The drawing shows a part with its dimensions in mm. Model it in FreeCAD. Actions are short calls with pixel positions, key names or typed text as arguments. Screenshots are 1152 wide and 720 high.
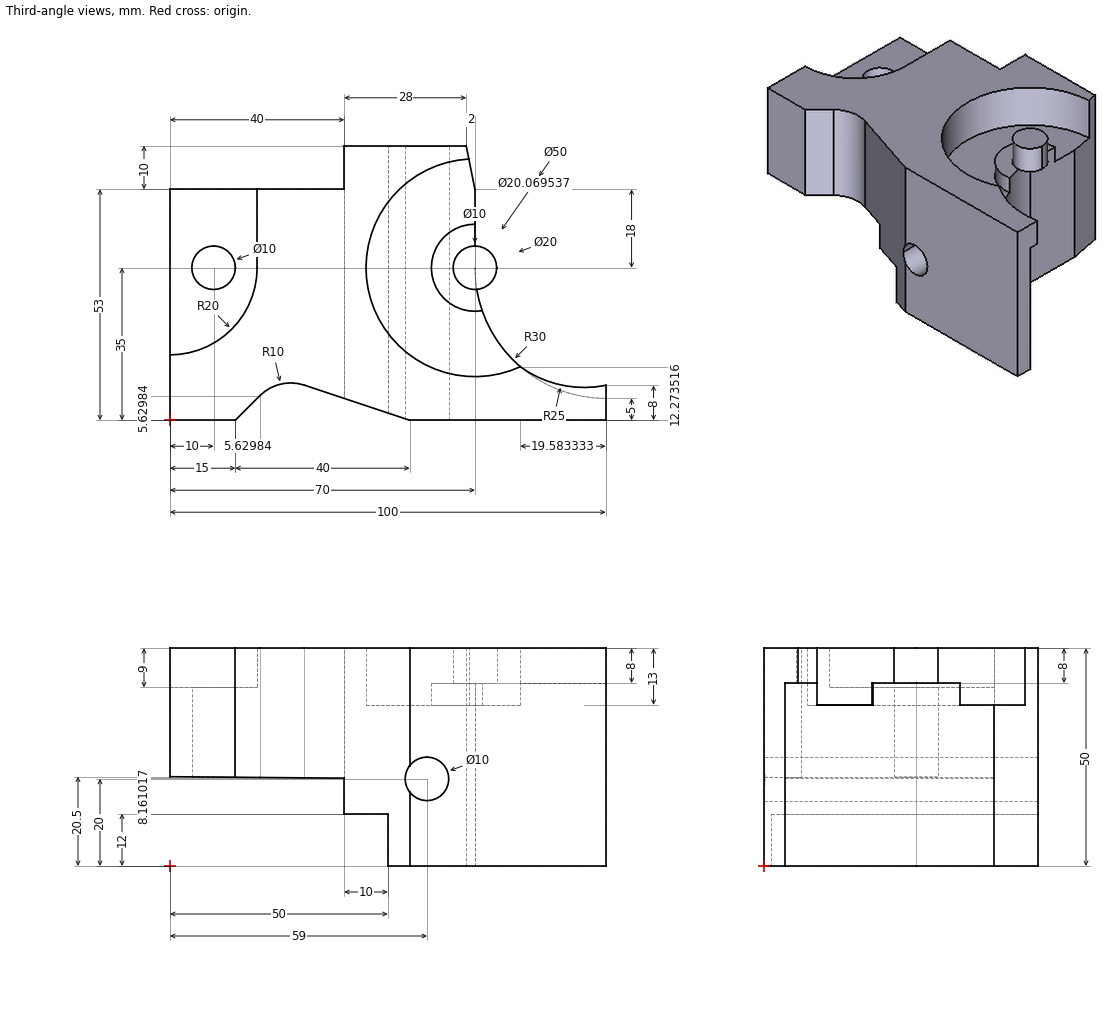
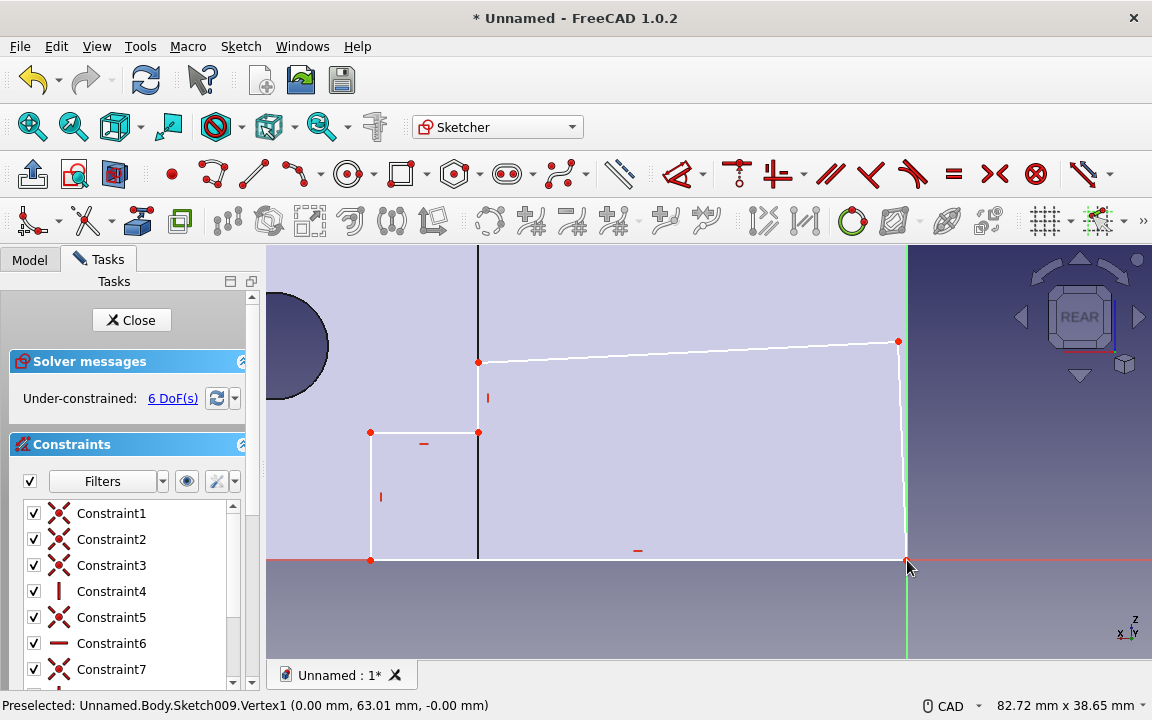
click(904, 495)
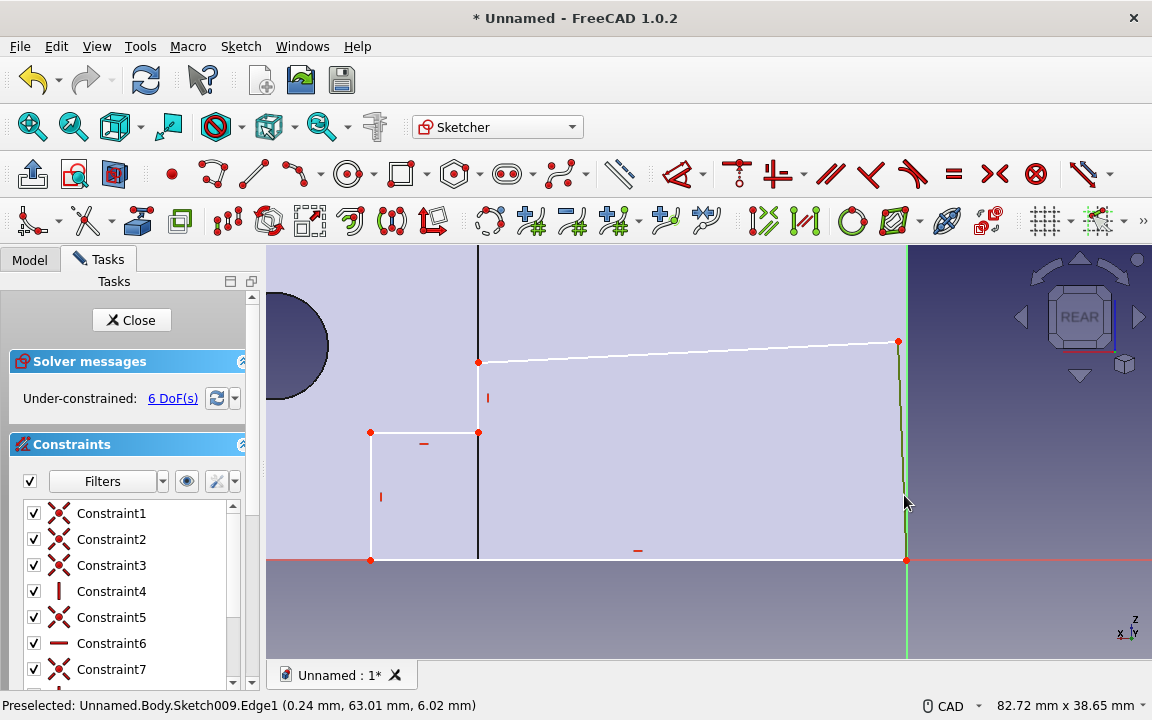
key(v)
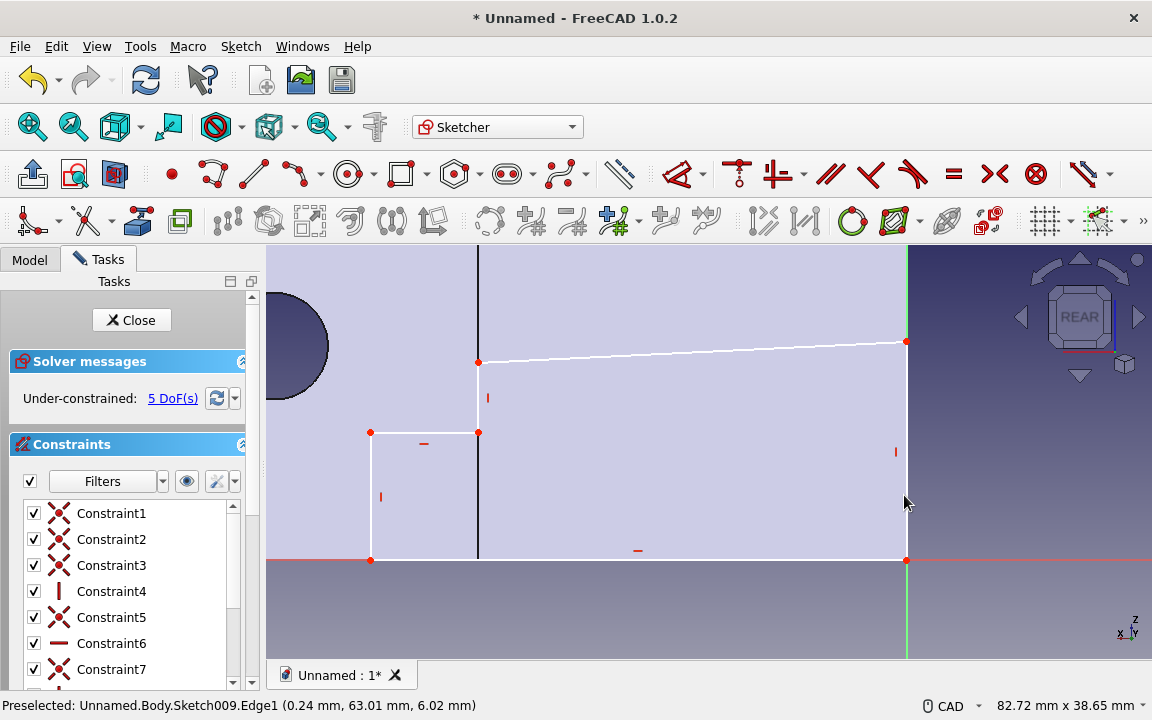
key(d)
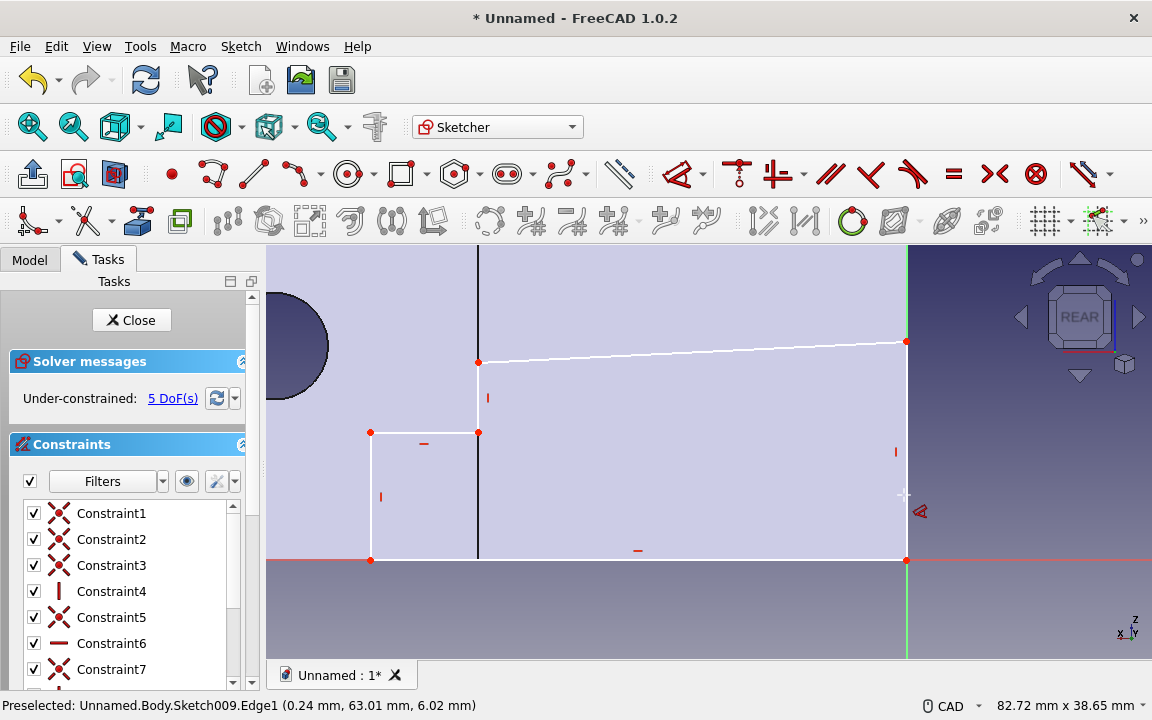
click(446, 433)
click(424, 399)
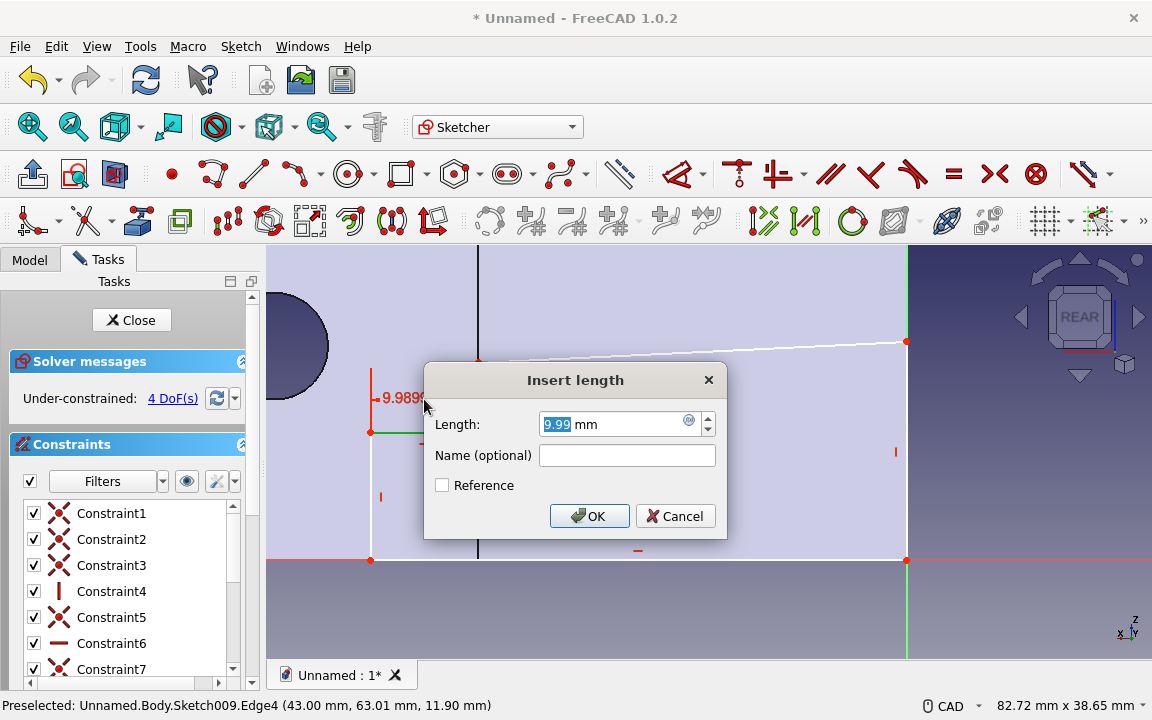
text(10)
key(Return)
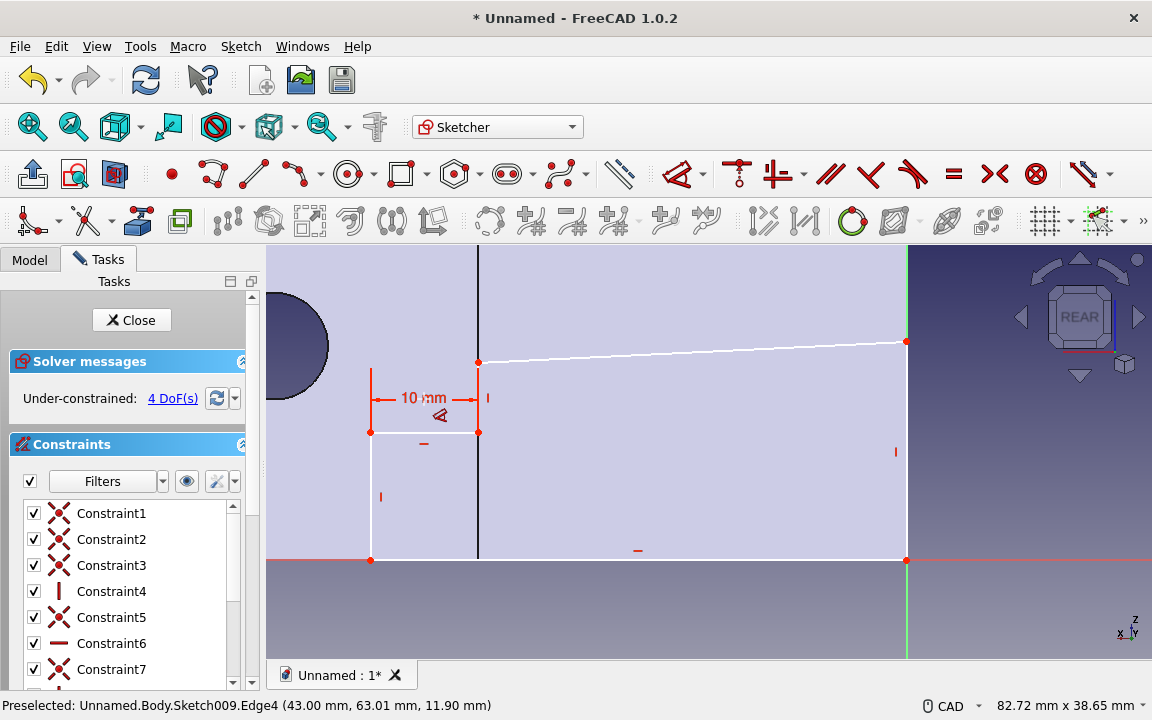
click(371, 471)
click(337, 497)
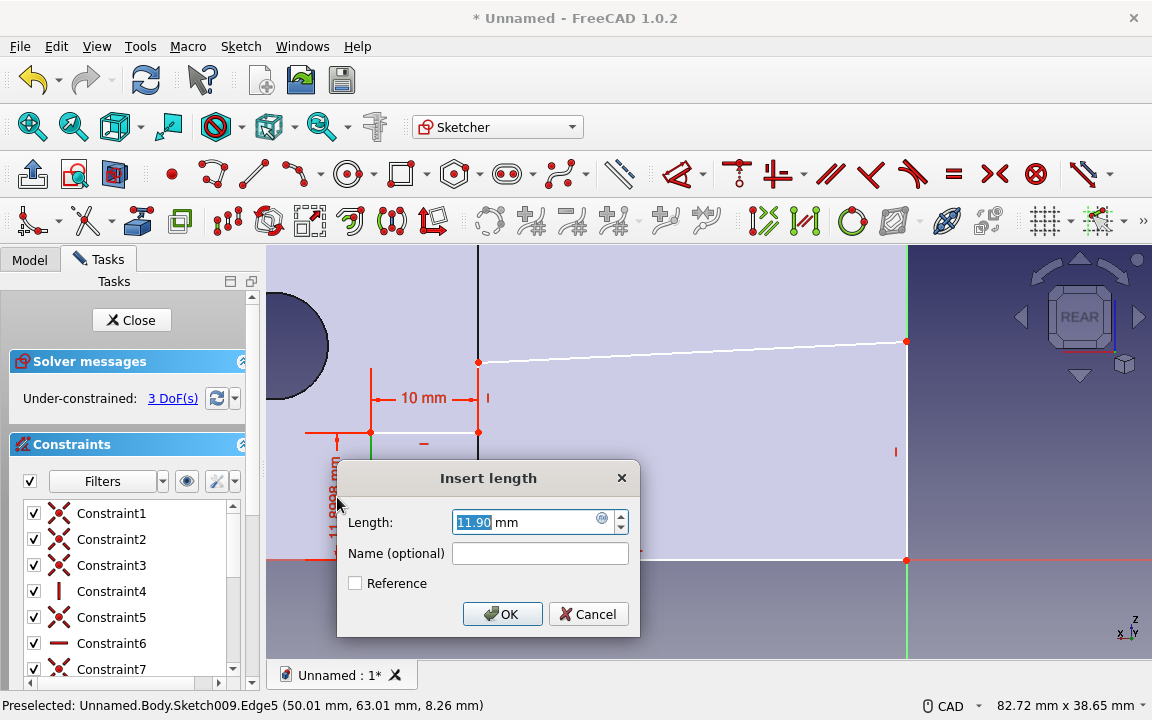
text(12)
key(Return)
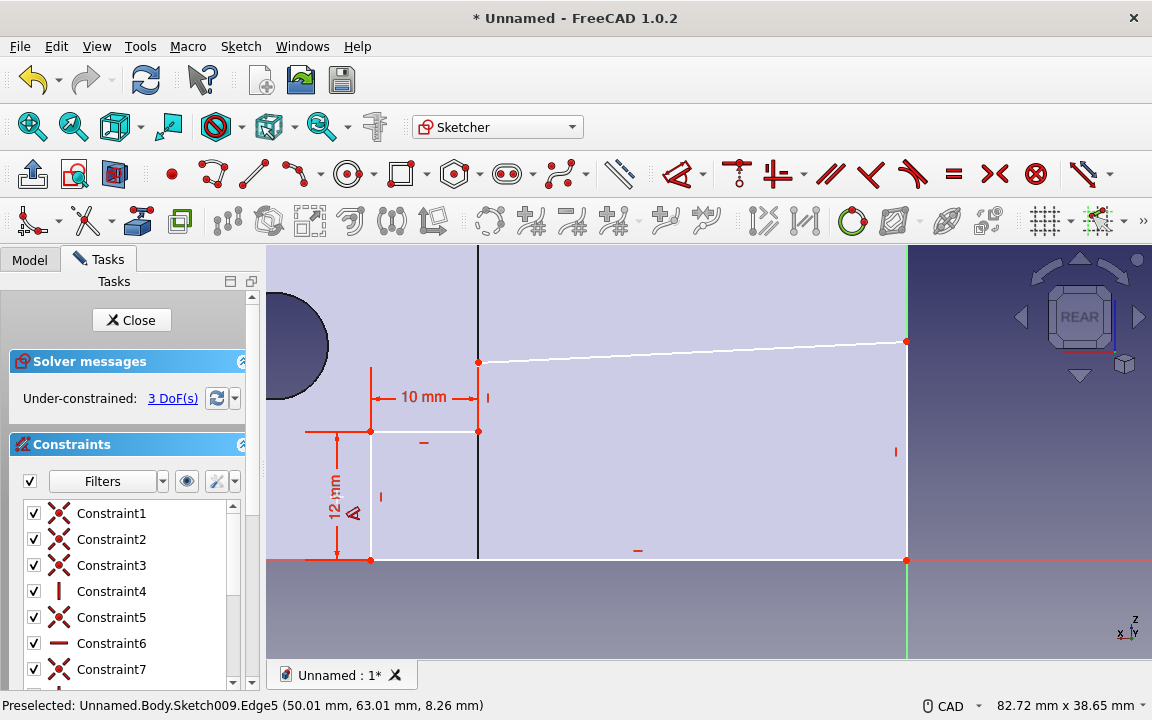
click(532, 560)
click(639, 594)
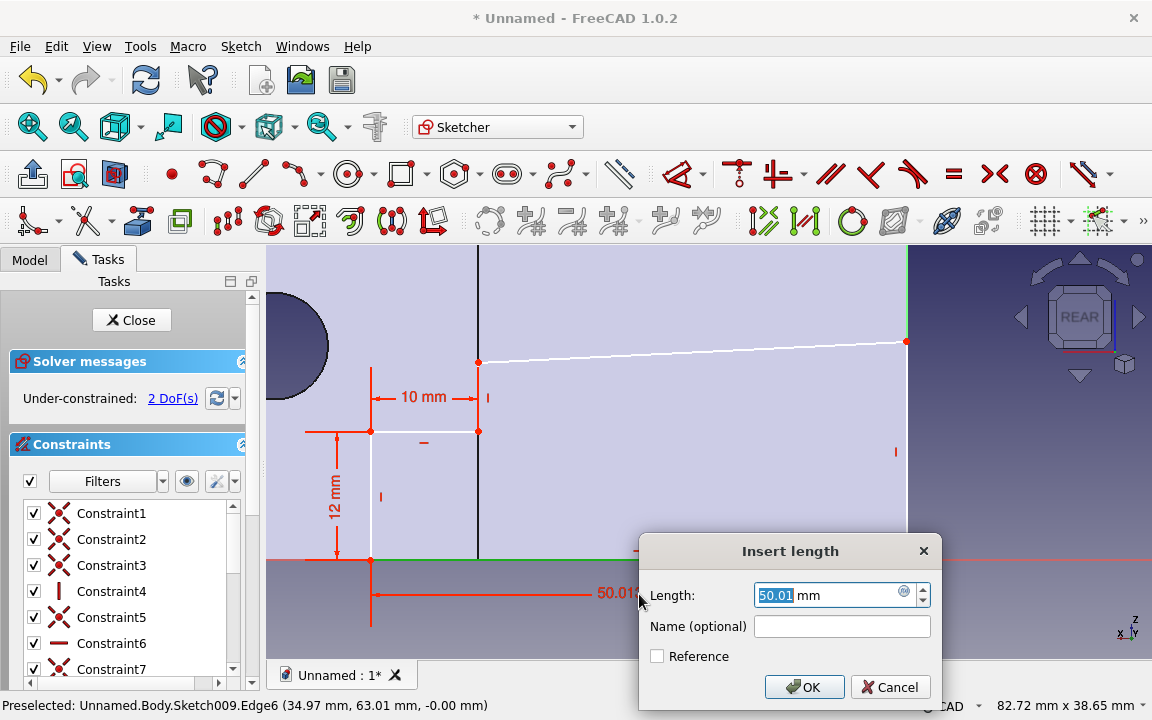
text(50)
key(Return)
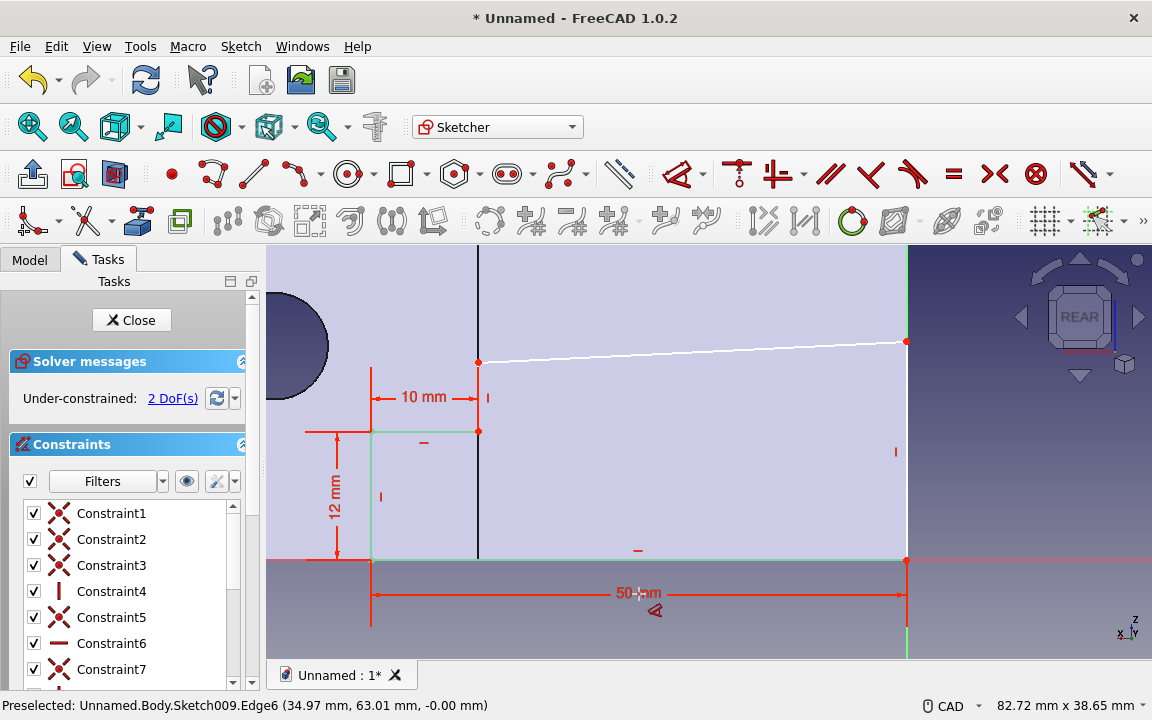
click(907, 495)
click(941, 451)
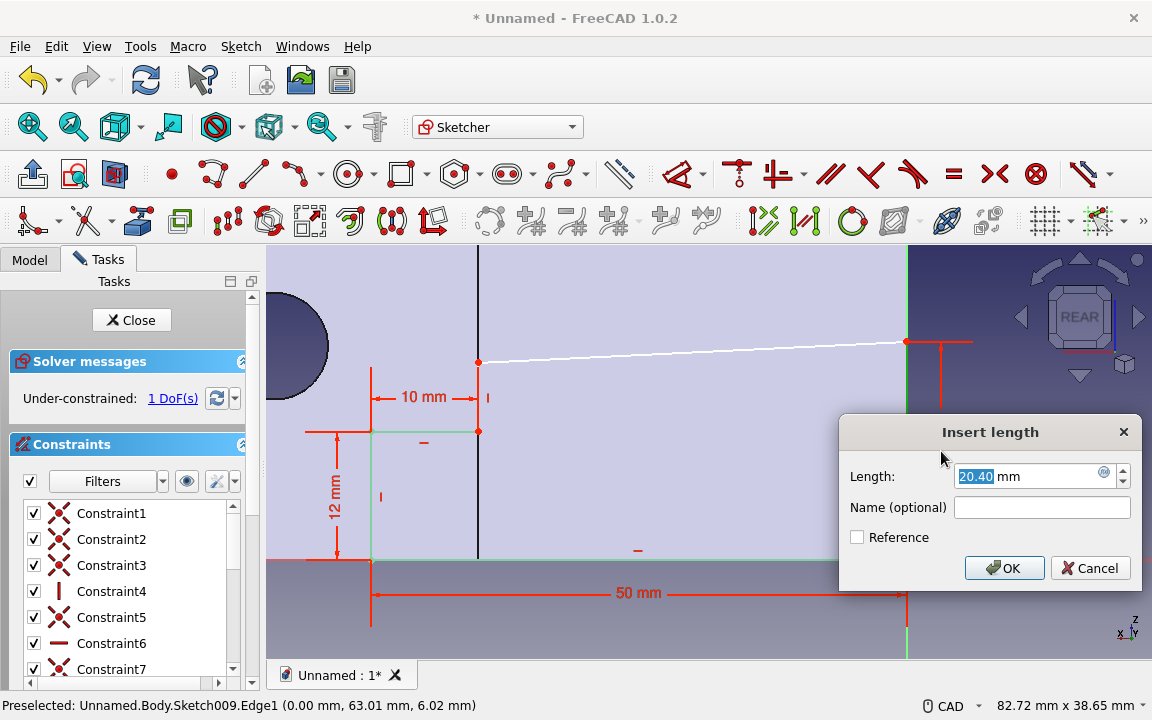
text(20.5)
key(Return)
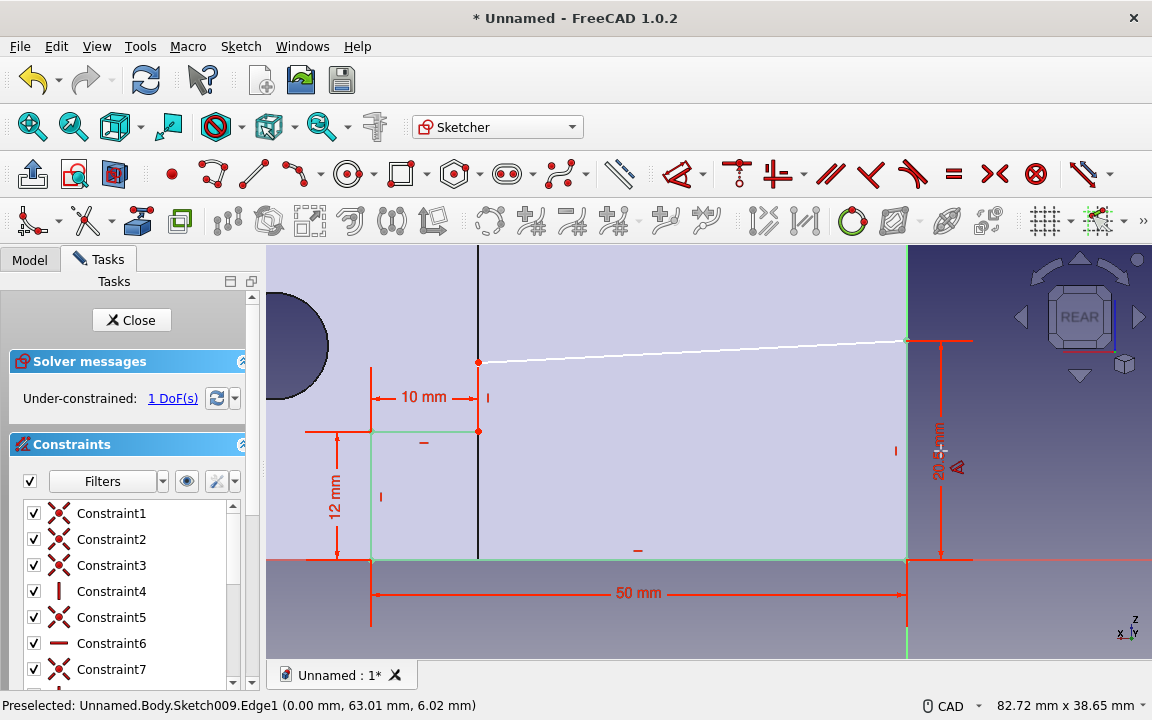
click(478, 384)
click(444, 373)